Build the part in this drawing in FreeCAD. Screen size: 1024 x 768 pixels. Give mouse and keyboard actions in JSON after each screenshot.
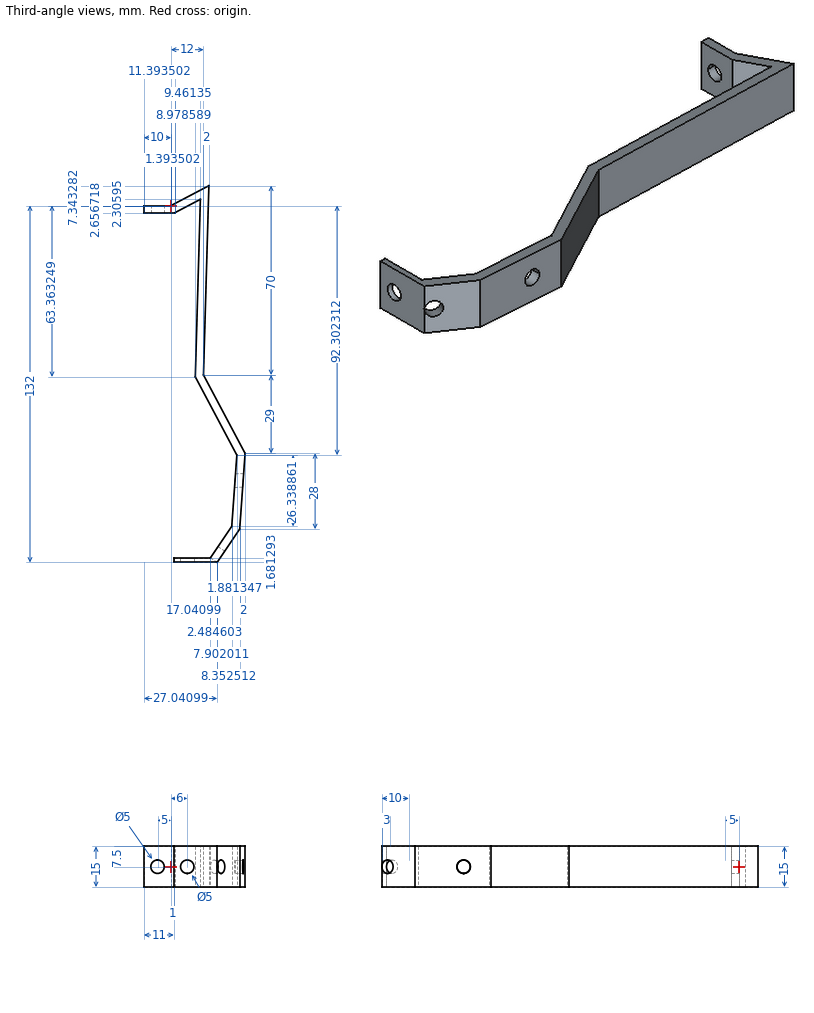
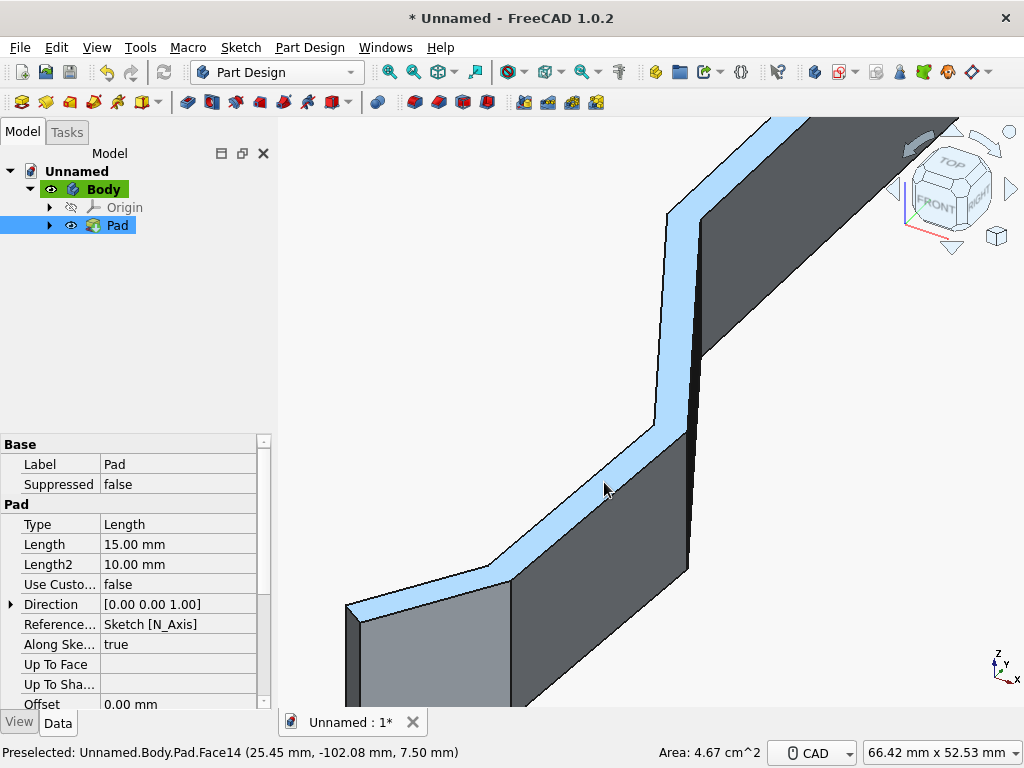
{"action": "left_click", "coordinate": [840, 72]}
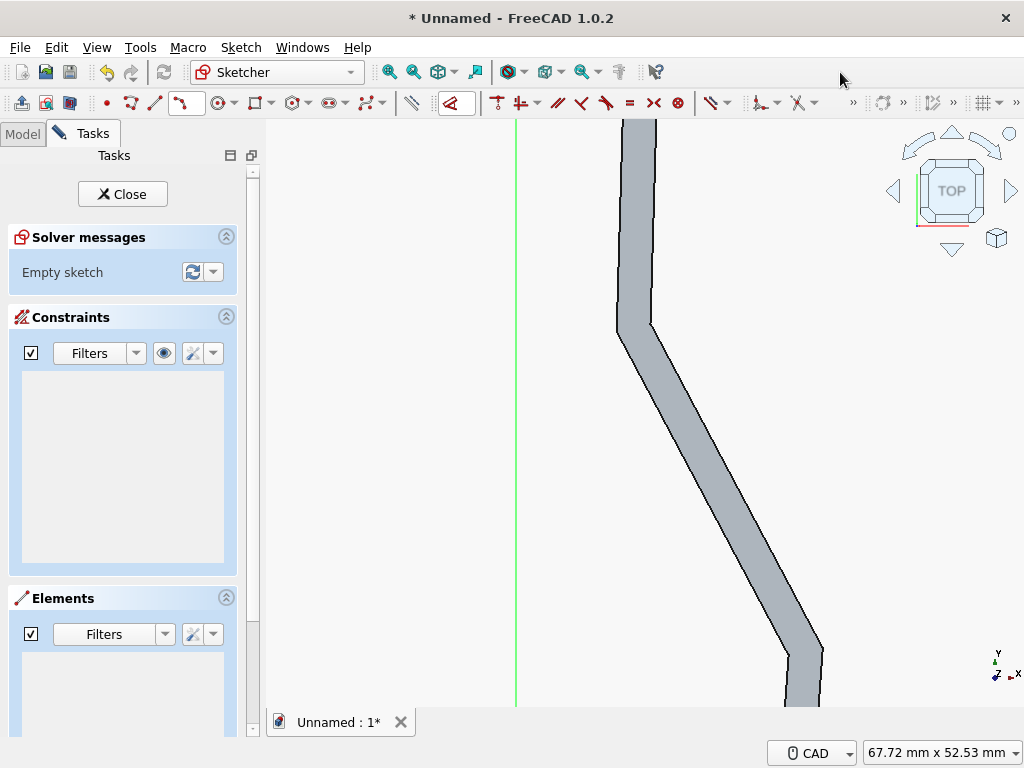
{"action": "scroll", "coordinate": [583, 430], "scroll_direction": "down", "scroll_amount": 7}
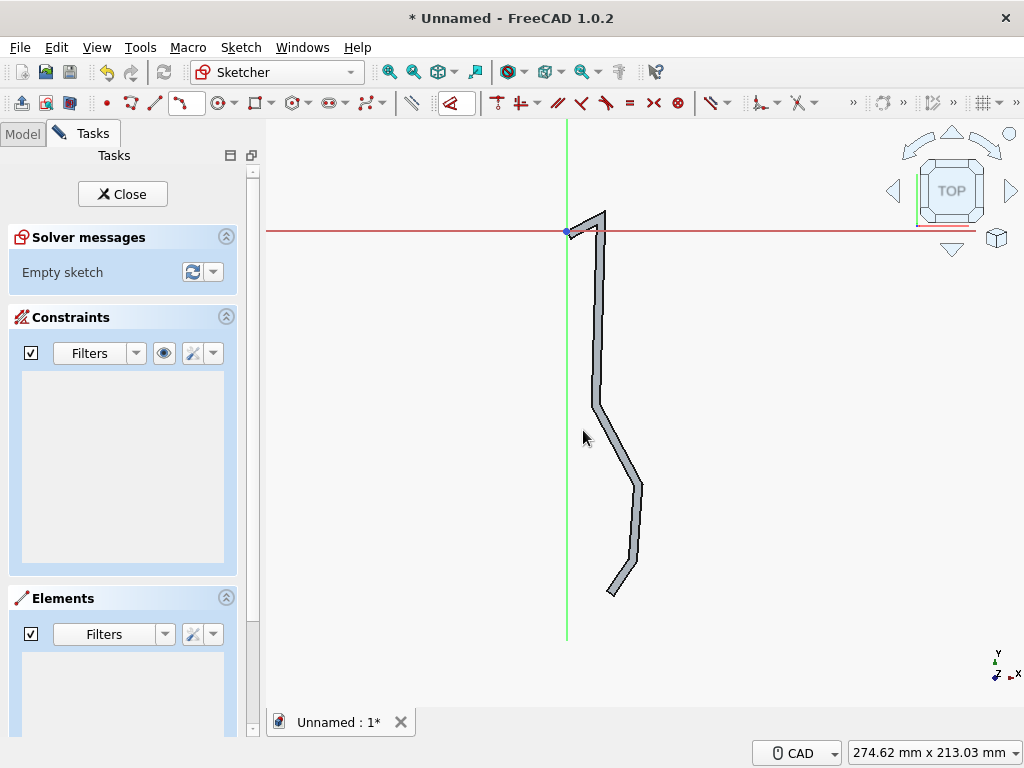
{"action": "left_click", "coordinate": [256, 104]}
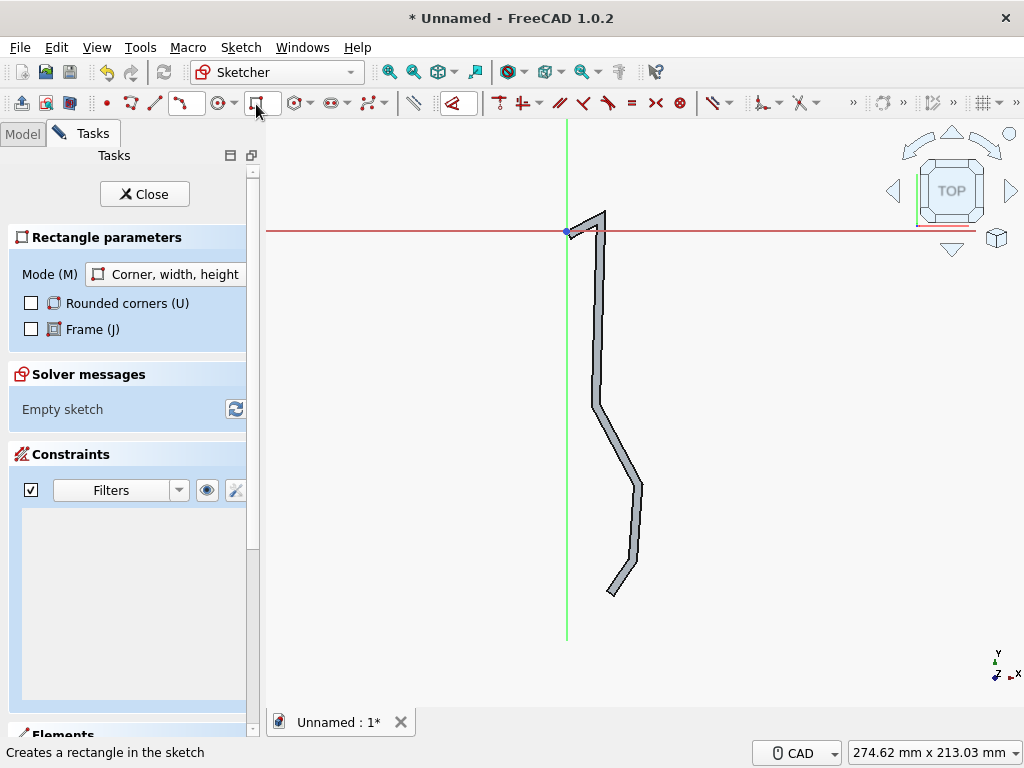
{"action": "scroll", "coordinate": [539, 231], "scroll_direction": "up", "scroll_amount": 4}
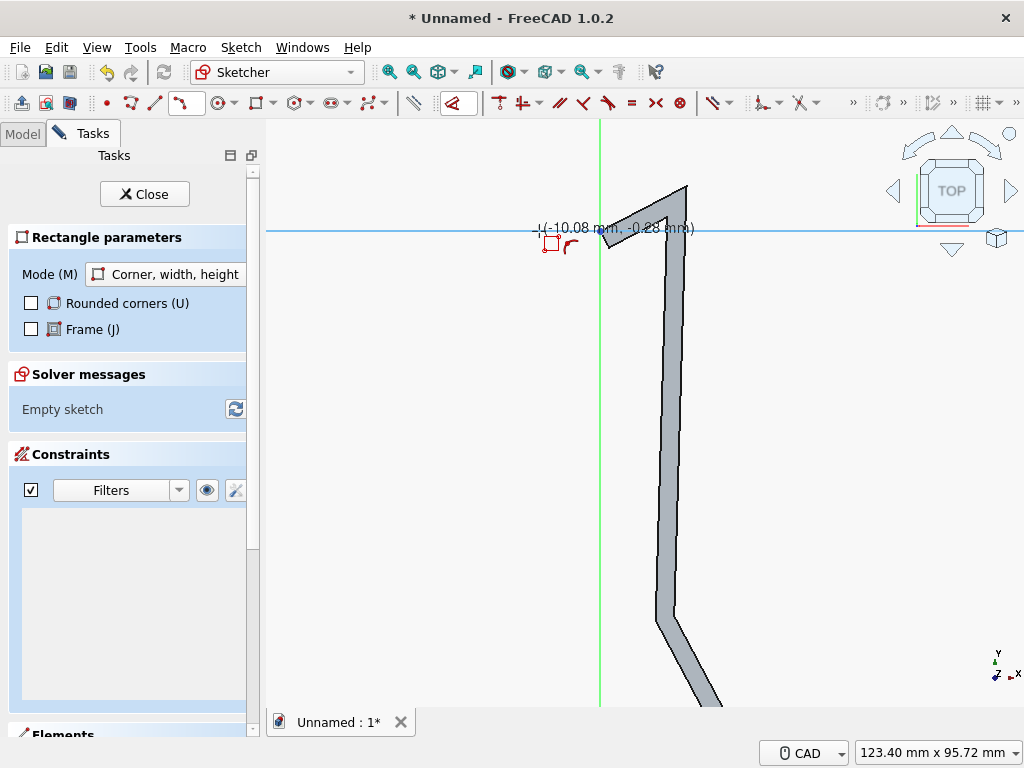
{"action": "left_click", "coordinate": [539, 231]}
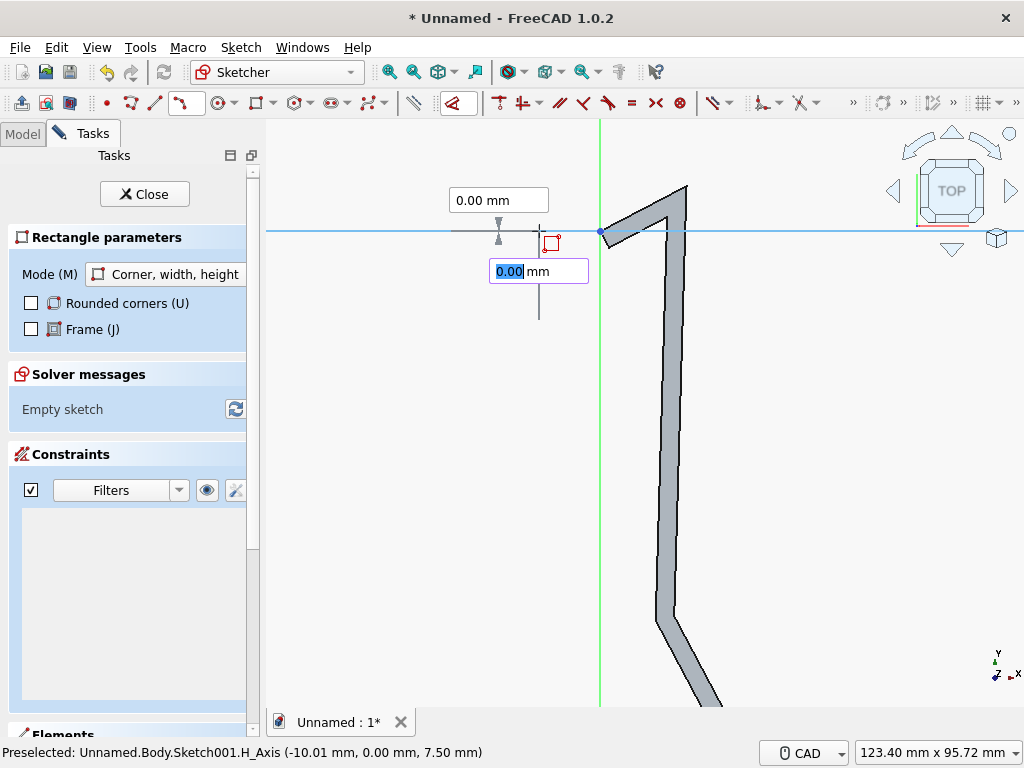
{"action": "scroll", "coordinate": [609, 248], "scroll_direction": "up", "scroll_amount": 4}
{"action": "mouse_move", "coordinate": [609, 247]}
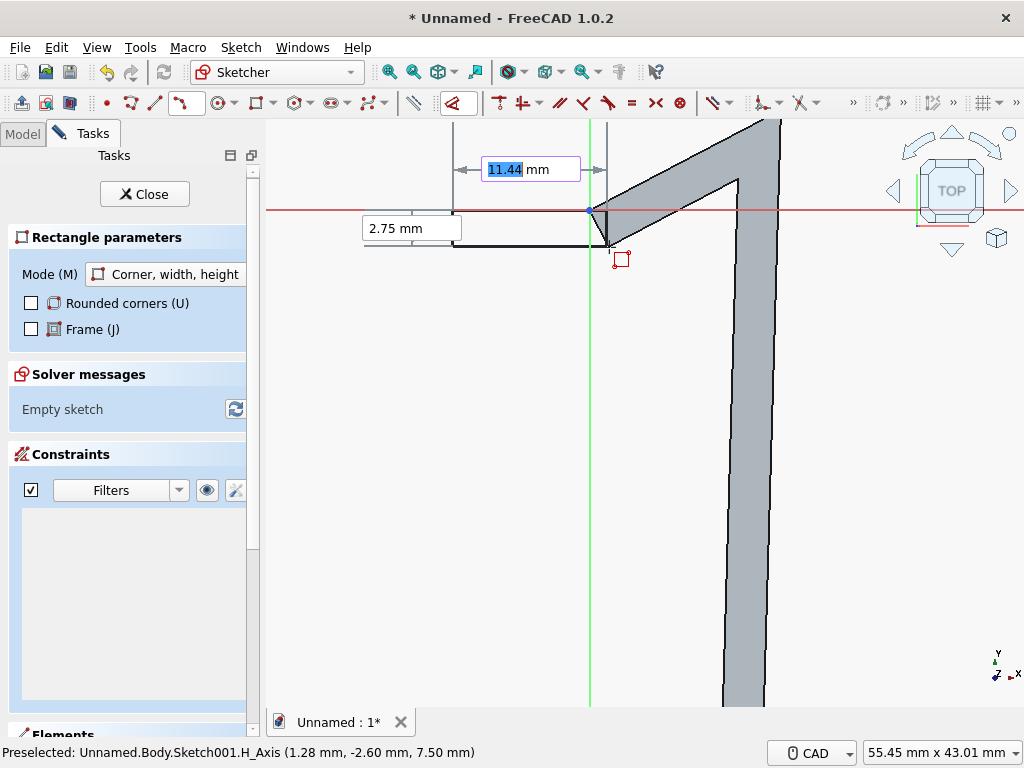
{"action": "type", "text": "11.393502"}
{"action": "key", "text": "Tab"}
{"action": "type", "text": "2.656718"}
{"action": "key", "text": "Return"}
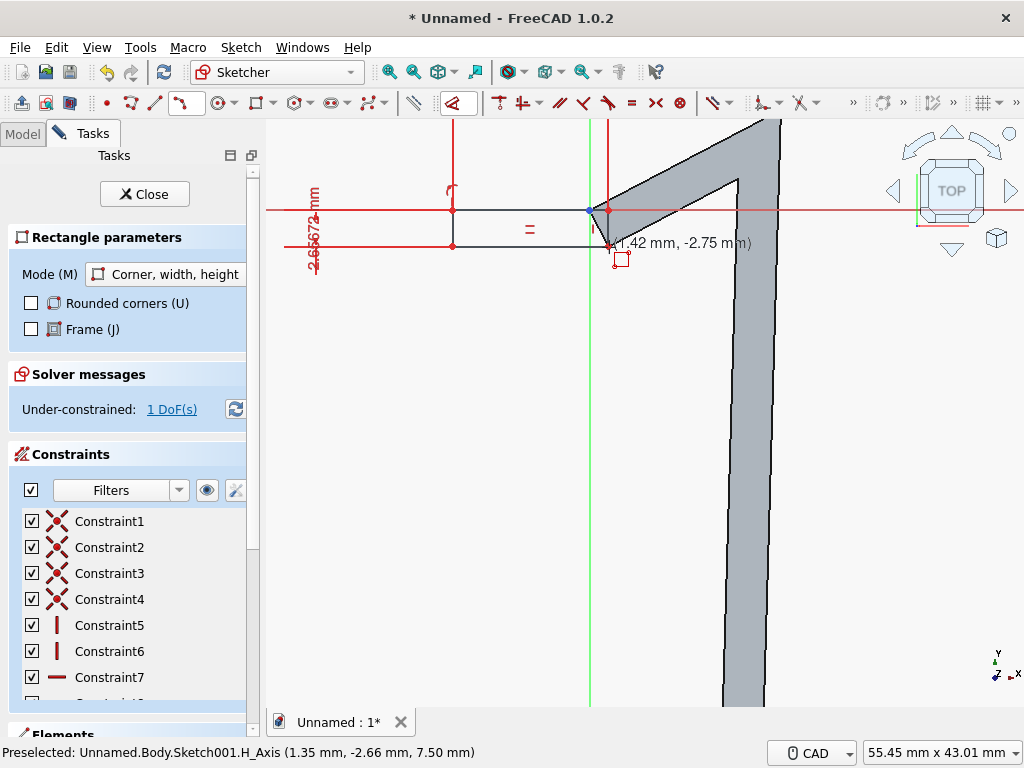
{"action": "scroll", "coordinate": [561, 236], "scroll_direction": "down", "scroll_amount": 8}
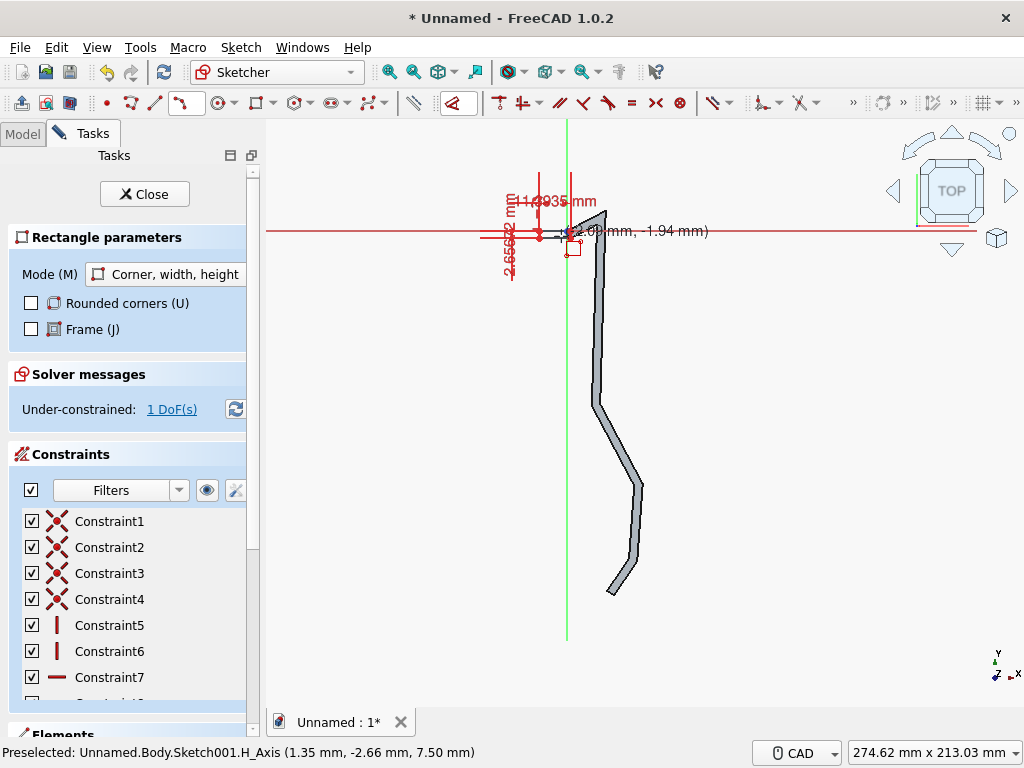
{"action": "scroll", "coordinate": [539, 591], "scroll_direction": "up", "scroll_amount": 7}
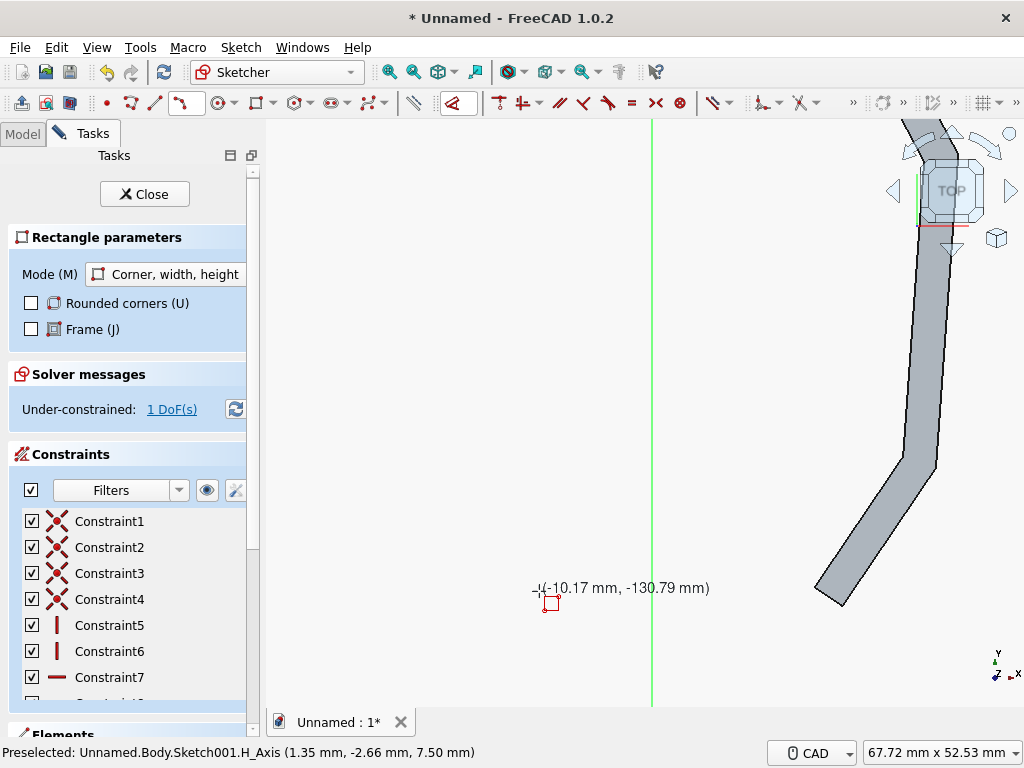
{"action": "scroll", "coordinate": [539, 592], "scroll_direction": "down", "scroll_amount": 7}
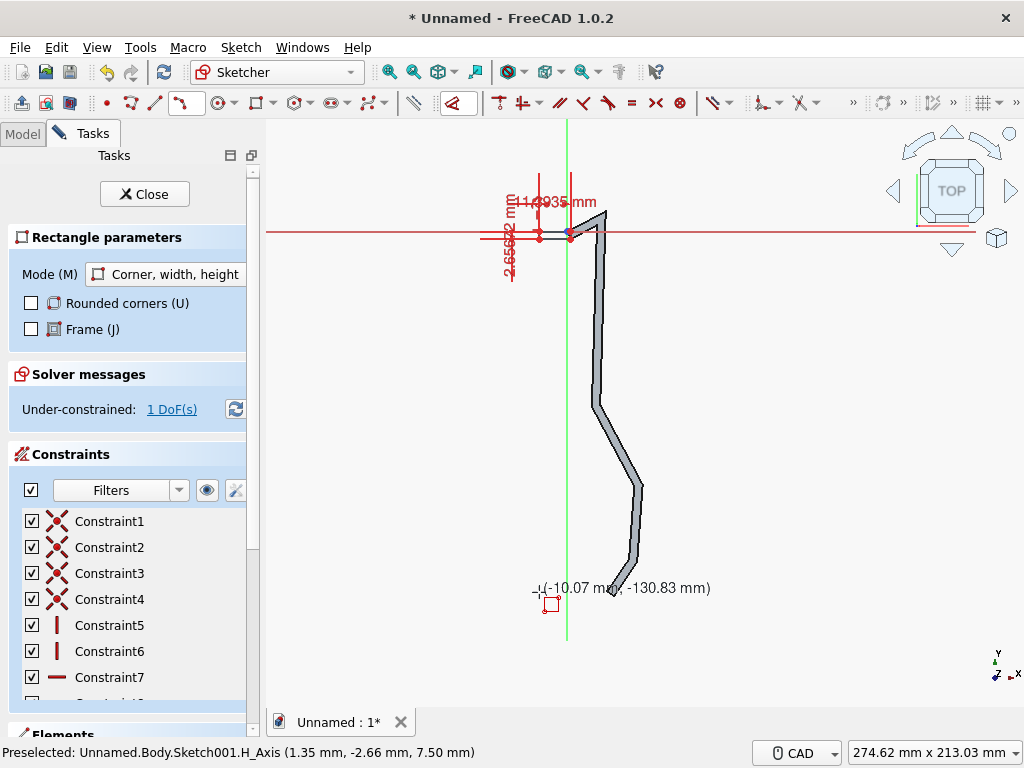
{"action": "left_click", "coordinate": [539, 591]}
{"action": "mouse_move", "coordinate": [614, 596]}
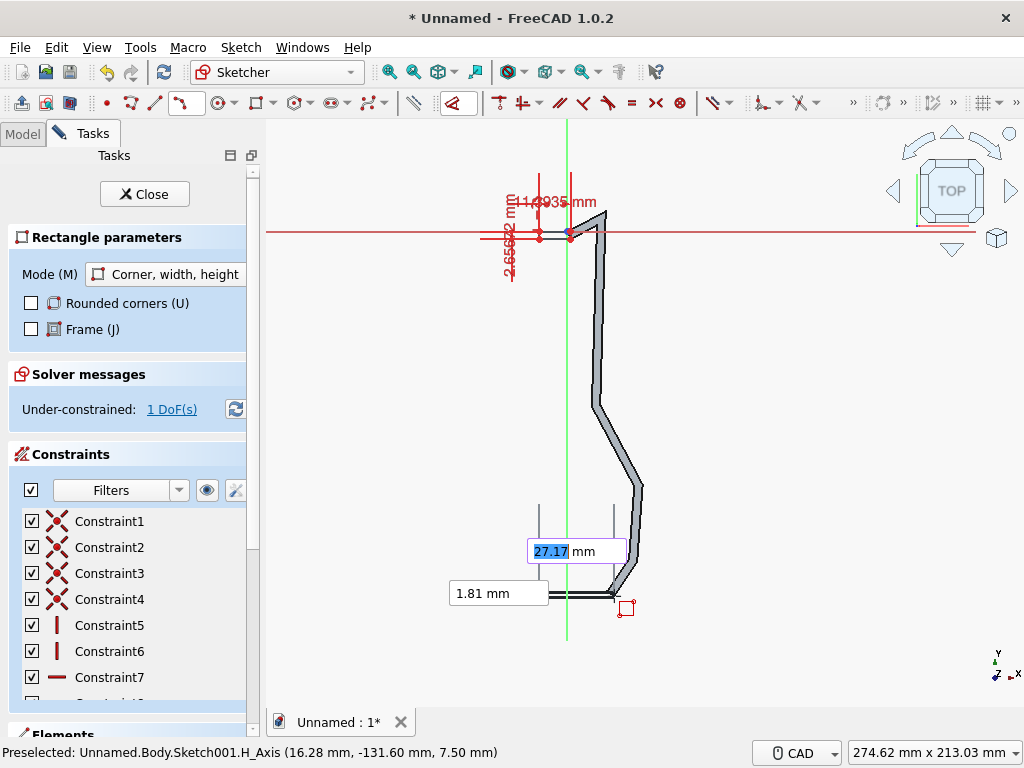
{"action": "type", "text": "27.04099"}
{"action": "key", "text": "Tab"}
{"action": "type", "text": "1.681293"}
{"action": "key", "text": "Return"}
{"action": "key", "text": "Escape"}